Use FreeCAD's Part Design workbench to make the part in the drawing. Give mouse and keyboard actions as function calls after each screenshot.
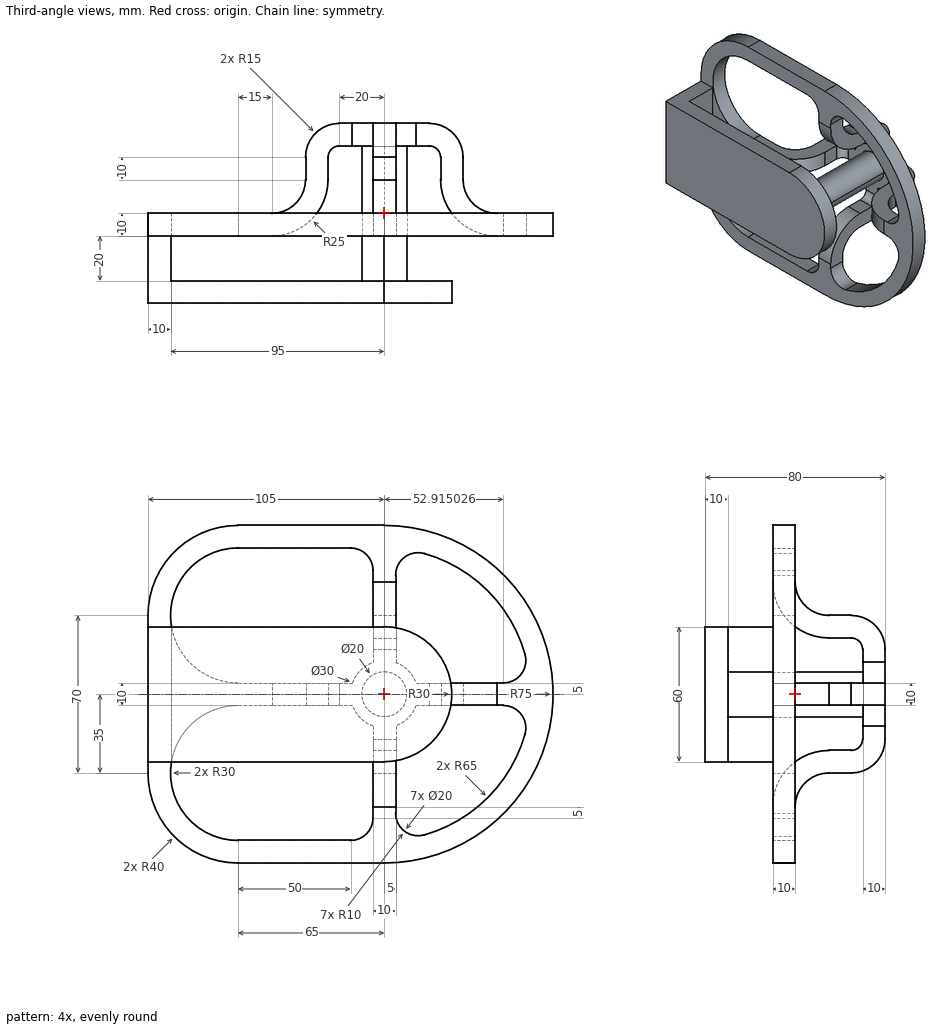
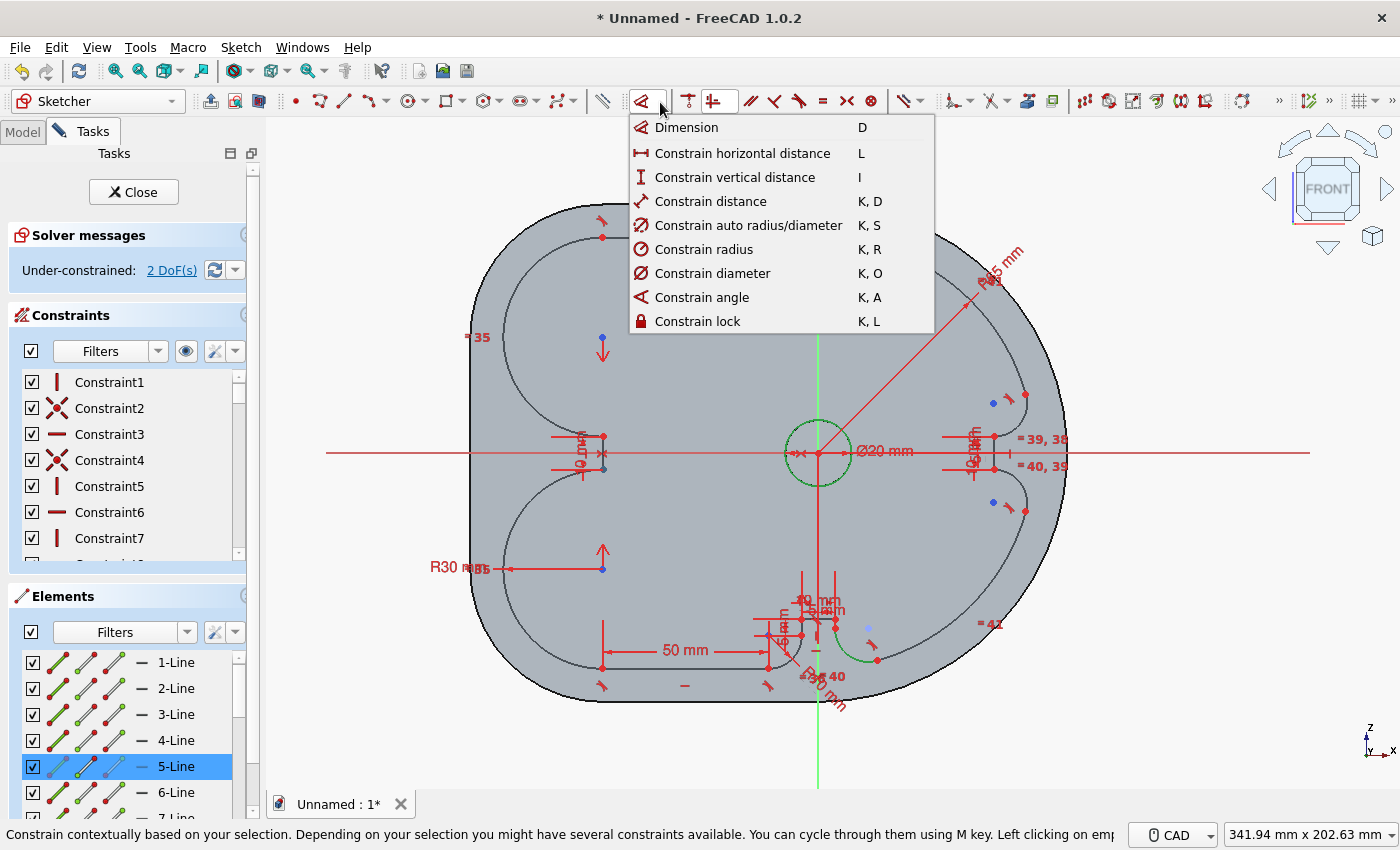
click(782, 153)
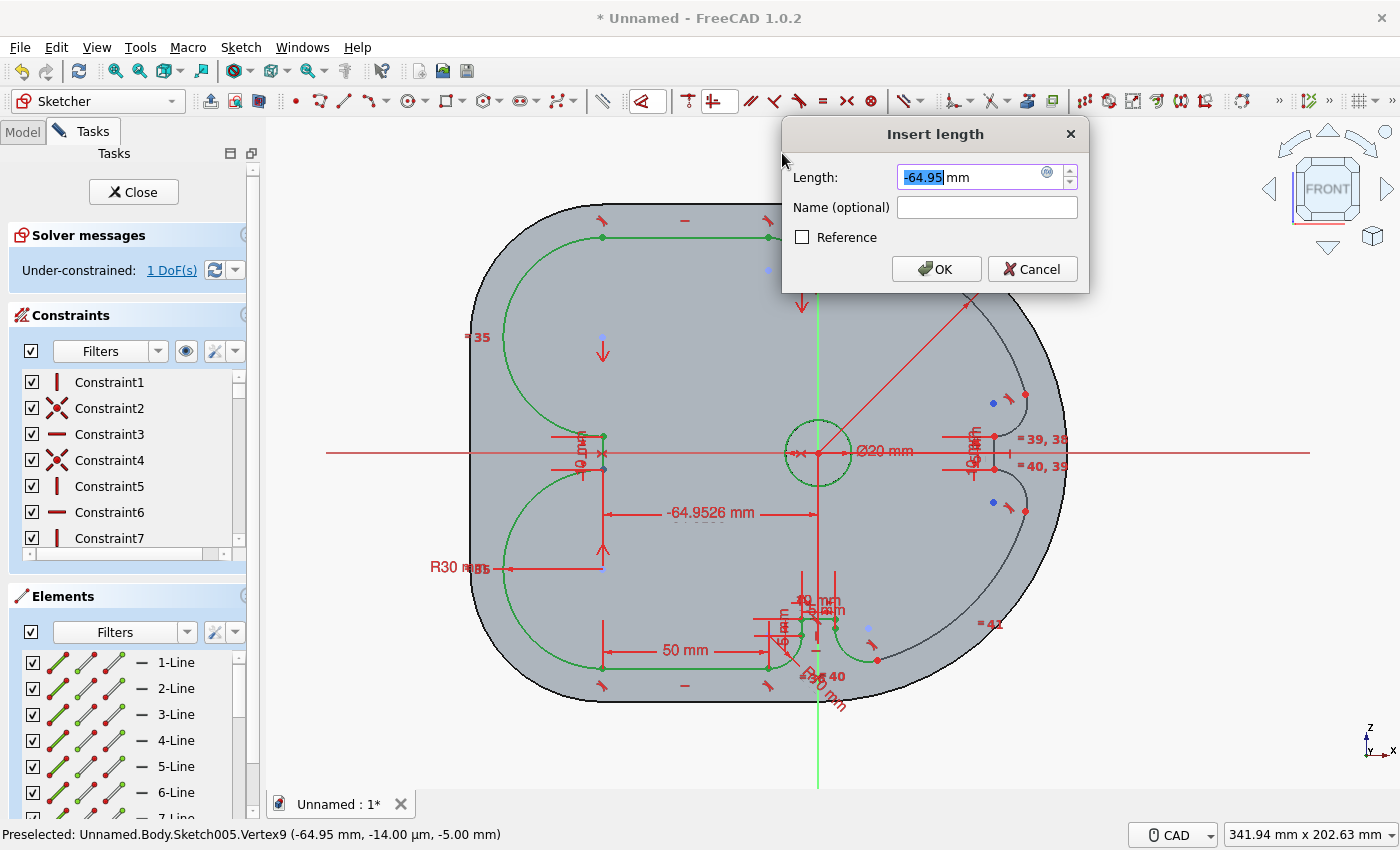
text(-65)
key(Return)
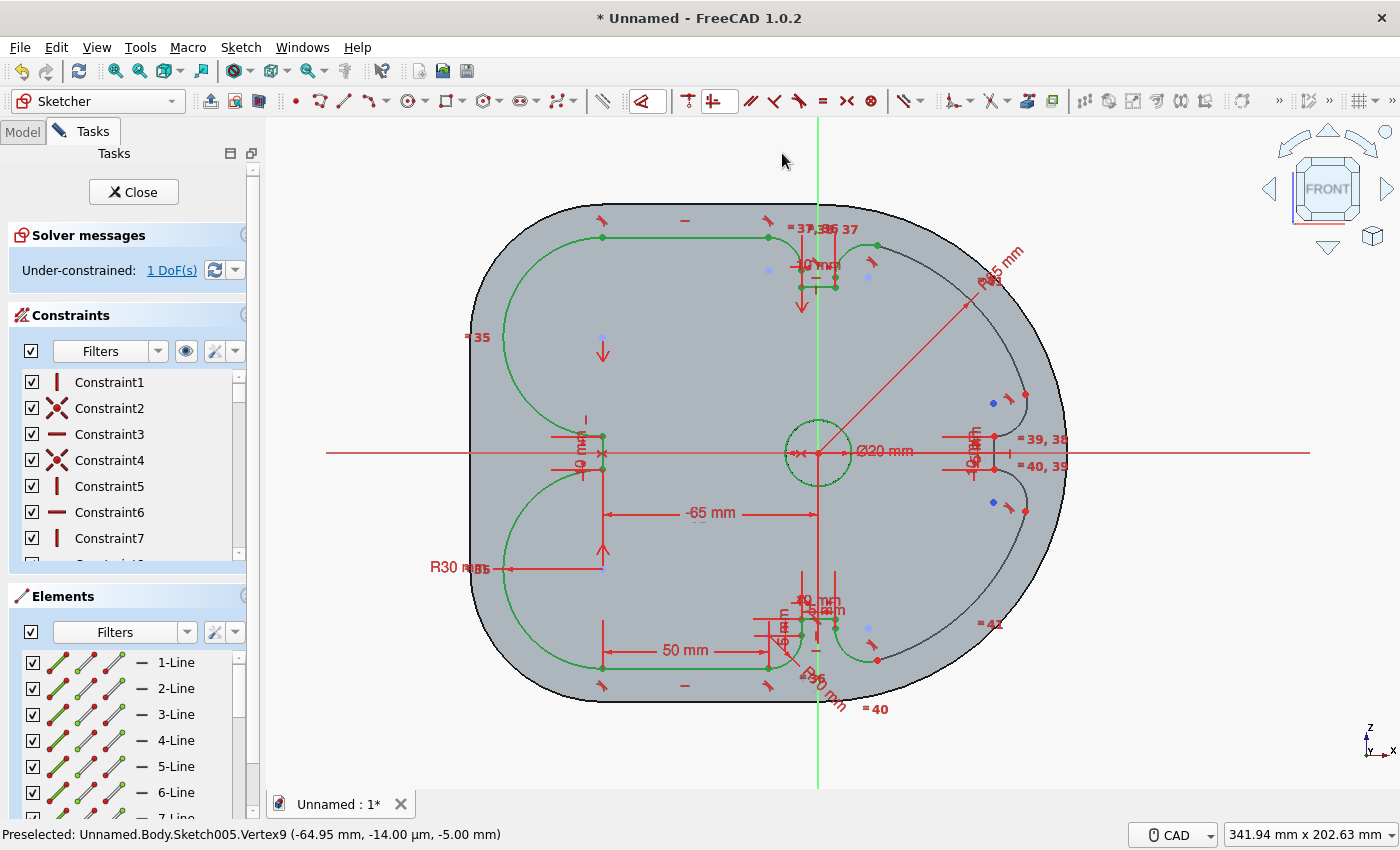
click(994, 437)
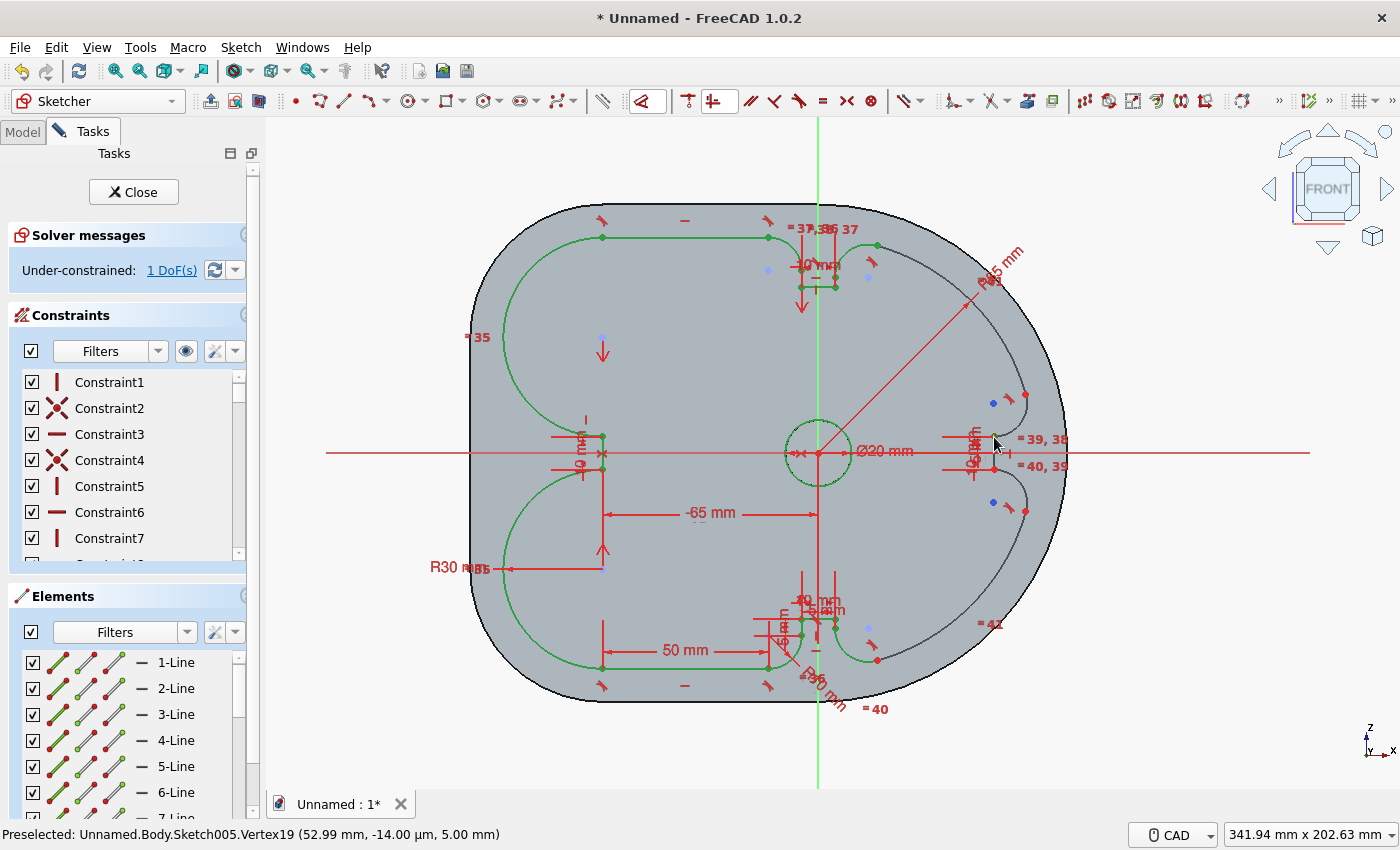
key(l)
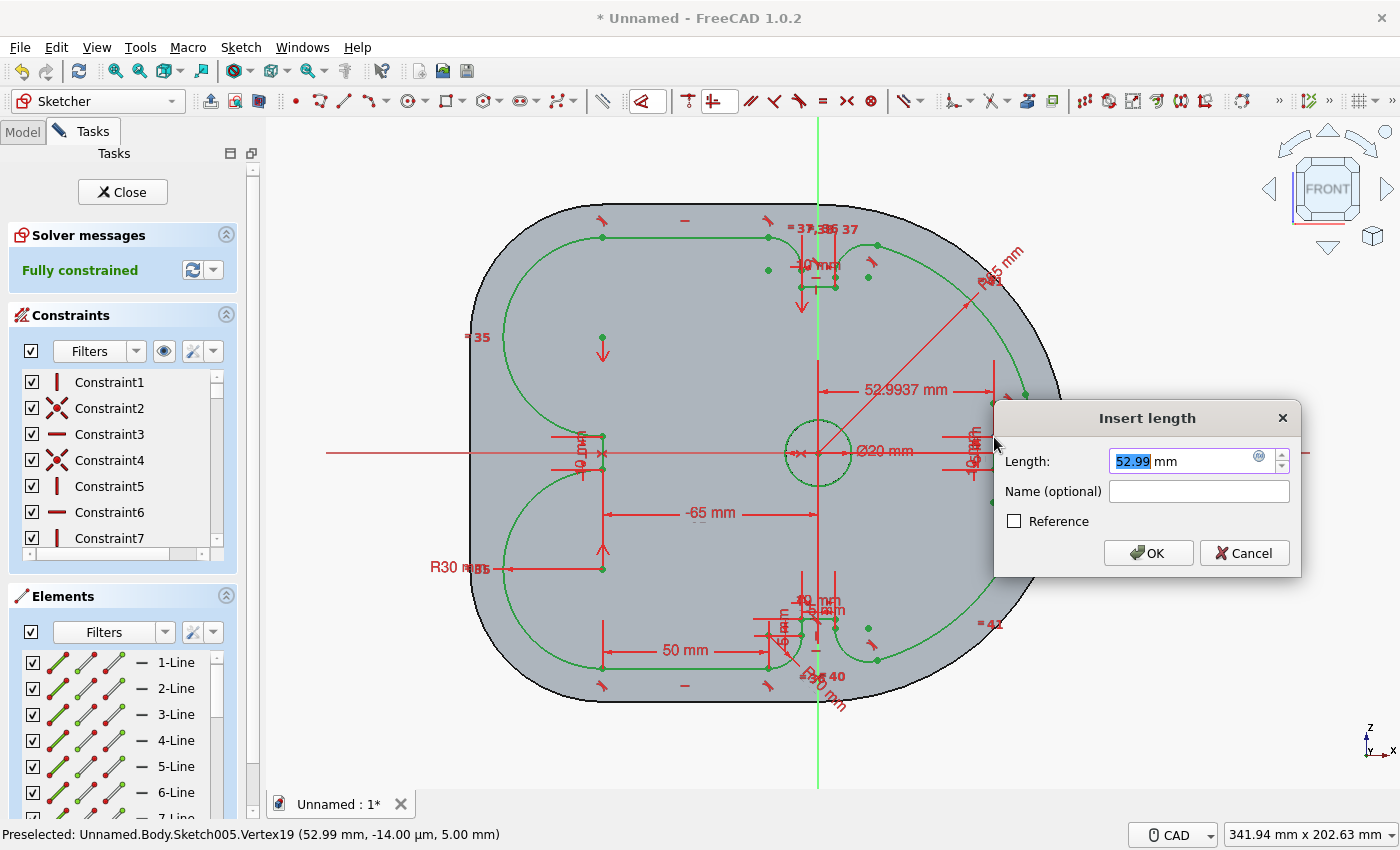
text(52.915026)
key(Return)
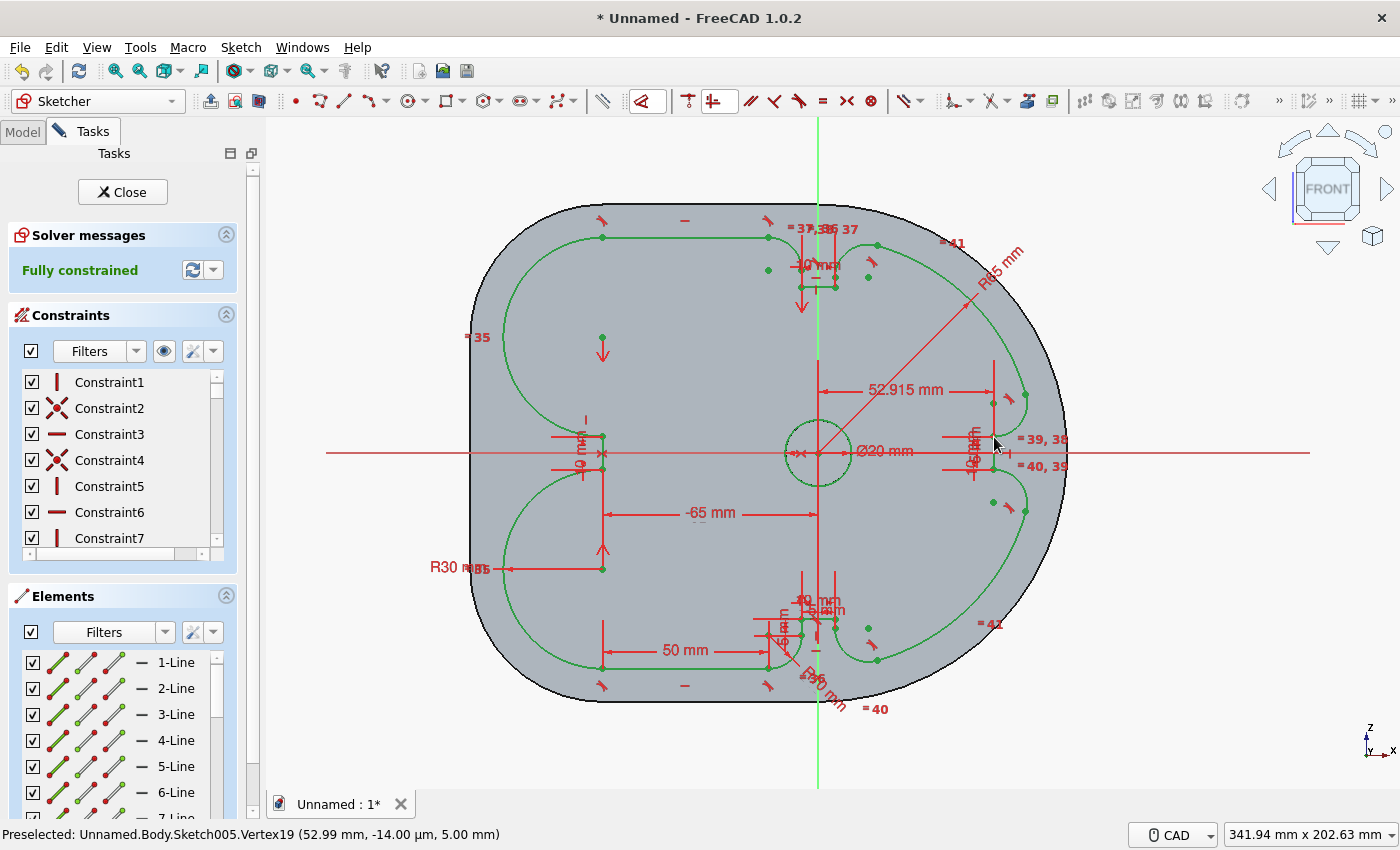
click(123, 192)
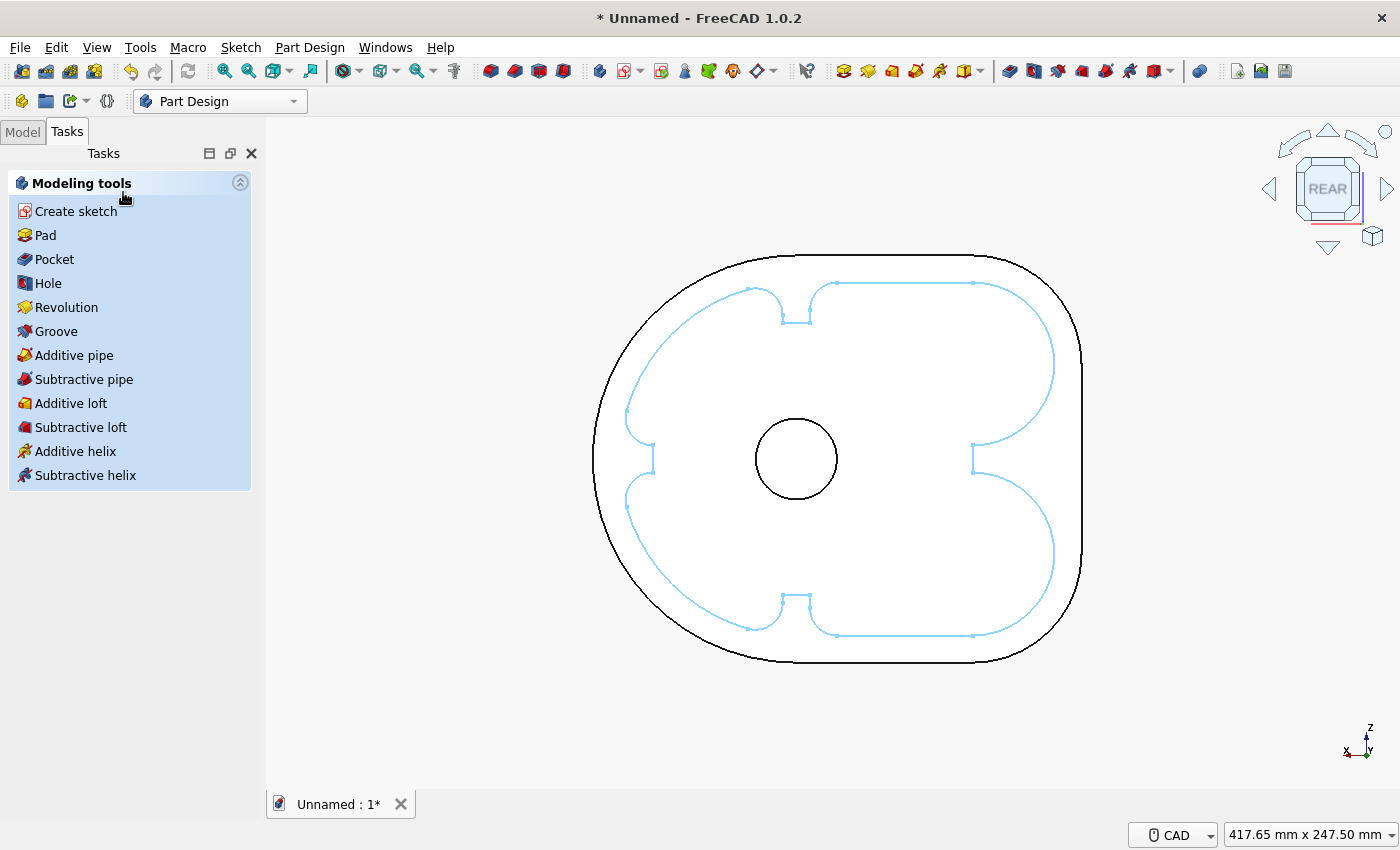
click(1010, 72)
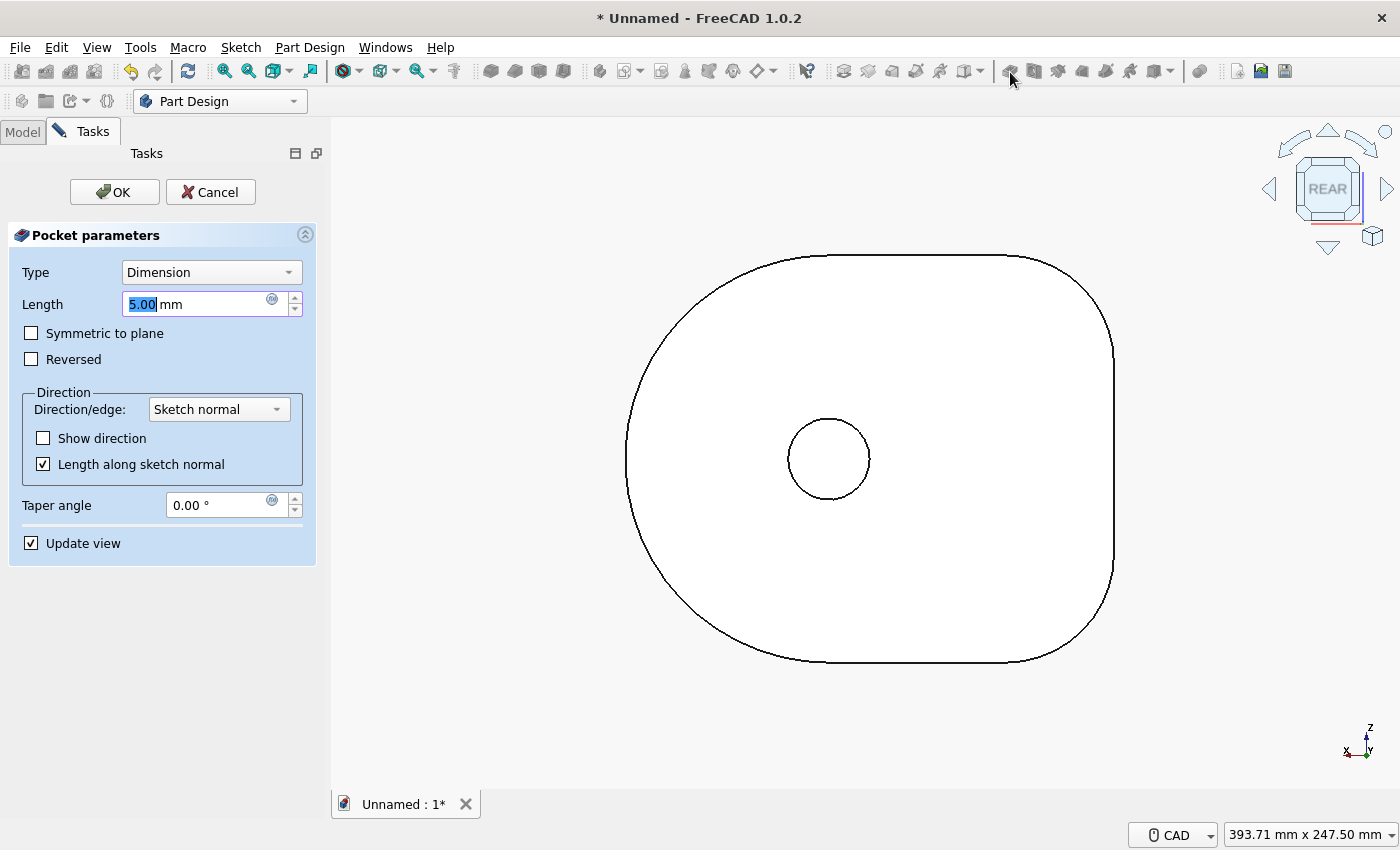
text(10)
key(Tab)